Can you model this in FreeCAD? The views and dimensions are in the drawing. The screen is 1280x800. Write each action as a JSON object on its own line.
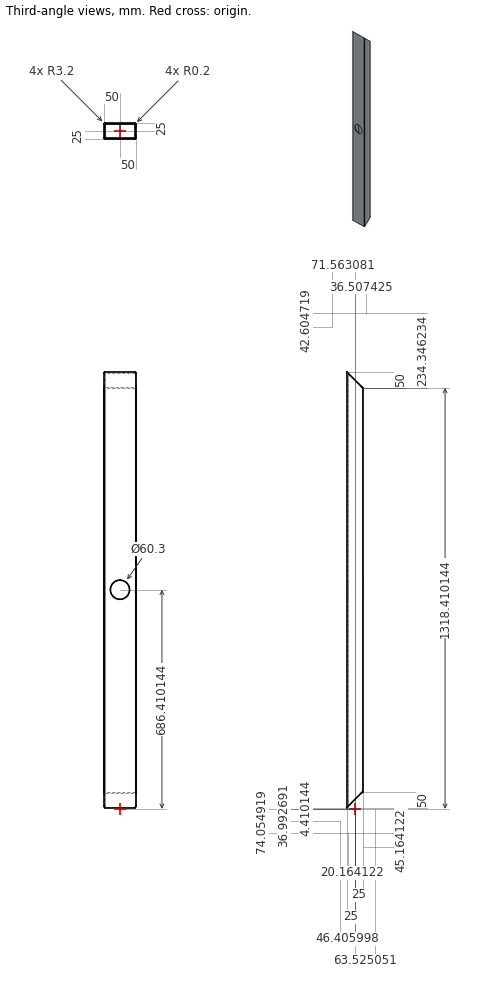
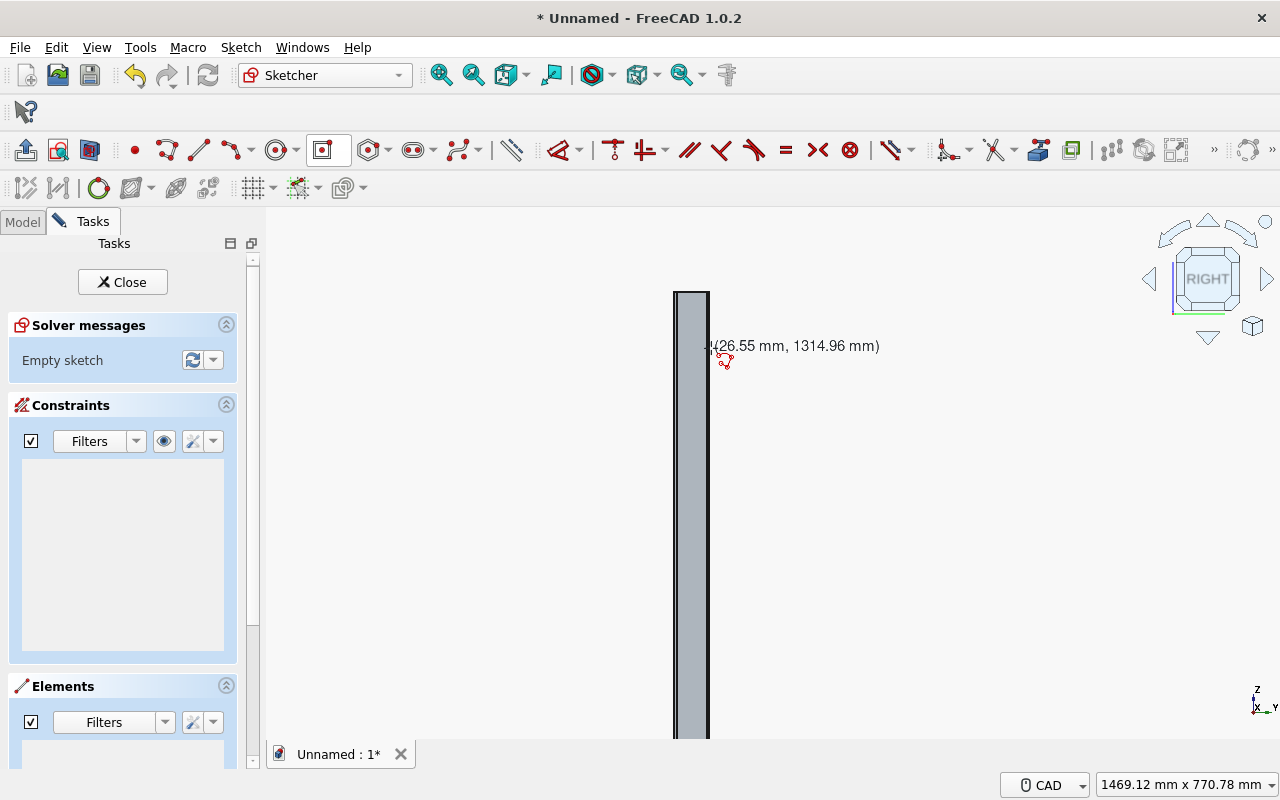
{"action": "left_click", "coordinate": [709, 348]}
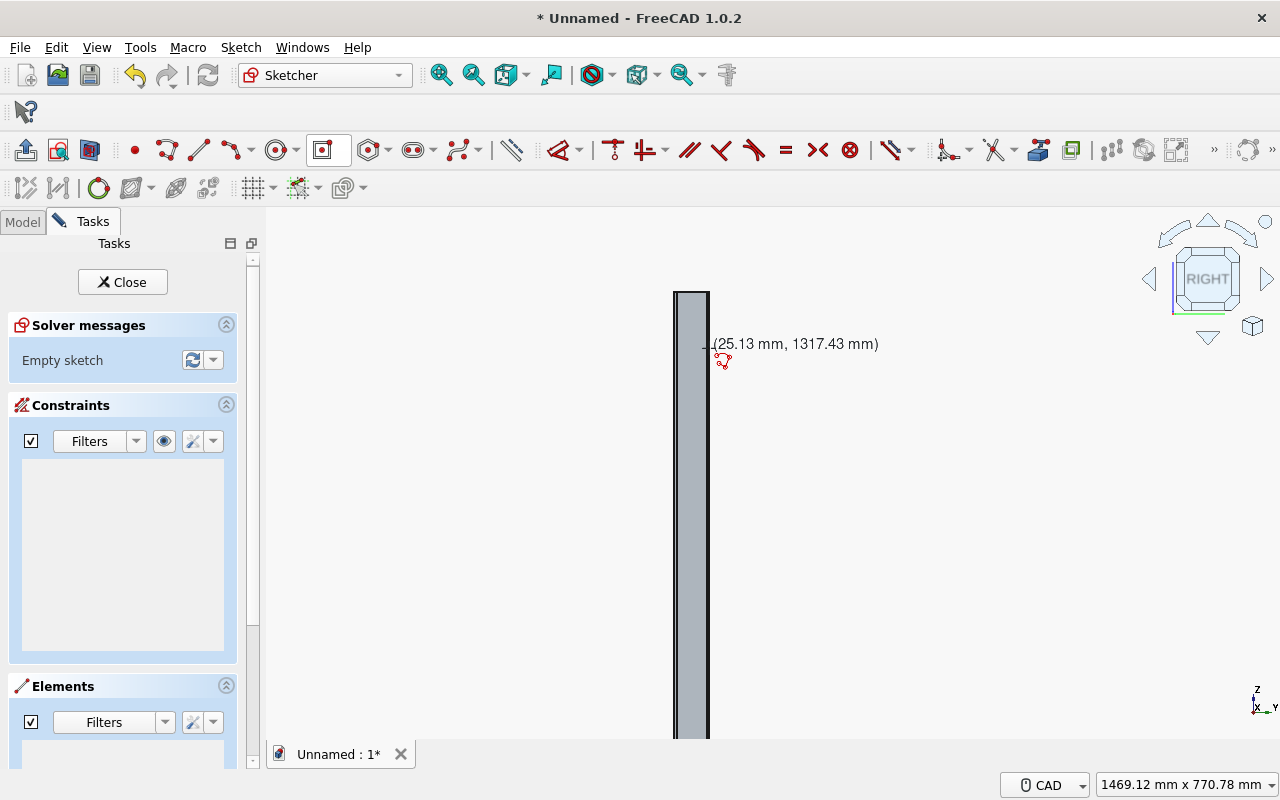
{"action": "scroll", "coordinate": [711, 348], "scroll_direction": "down", "scroll_amount": 6}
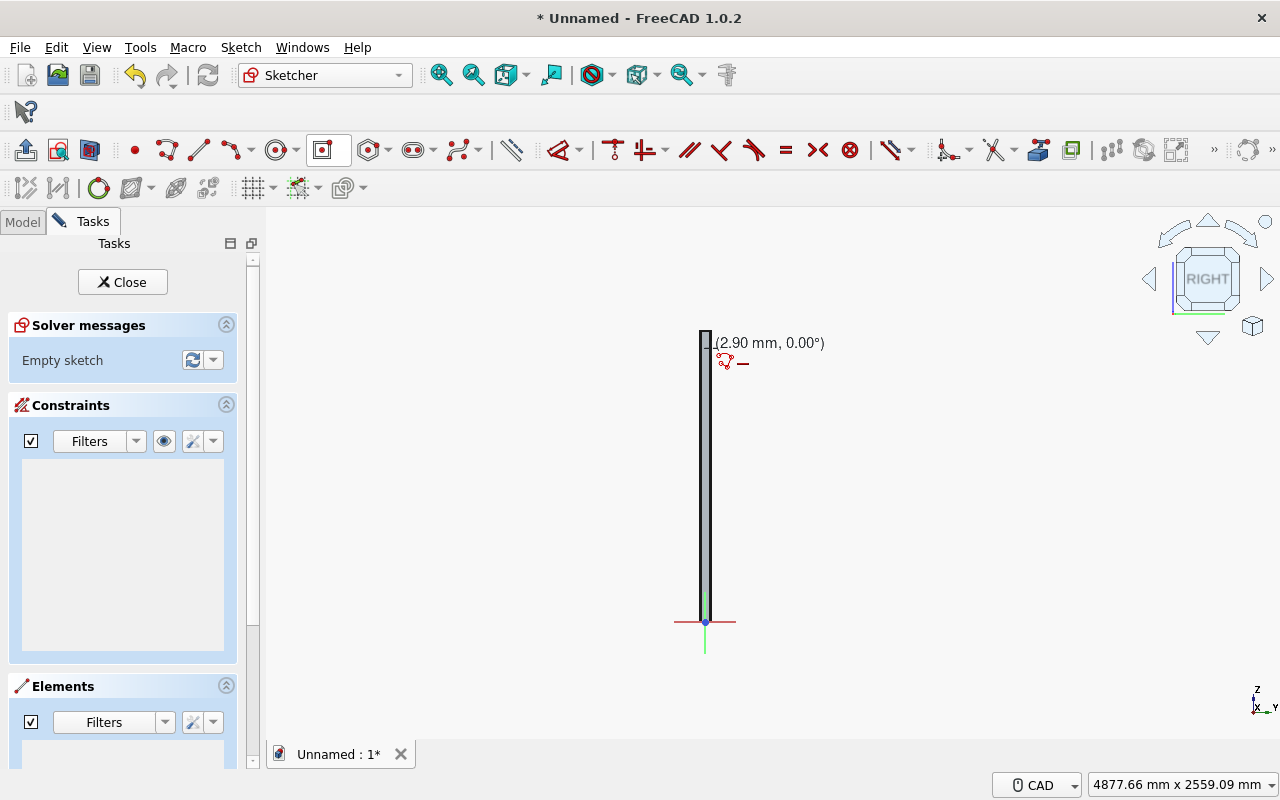
{"action": "scroll", "coordinate": [713, 300], "scroll_direction": "up", "scroll_amount": 4}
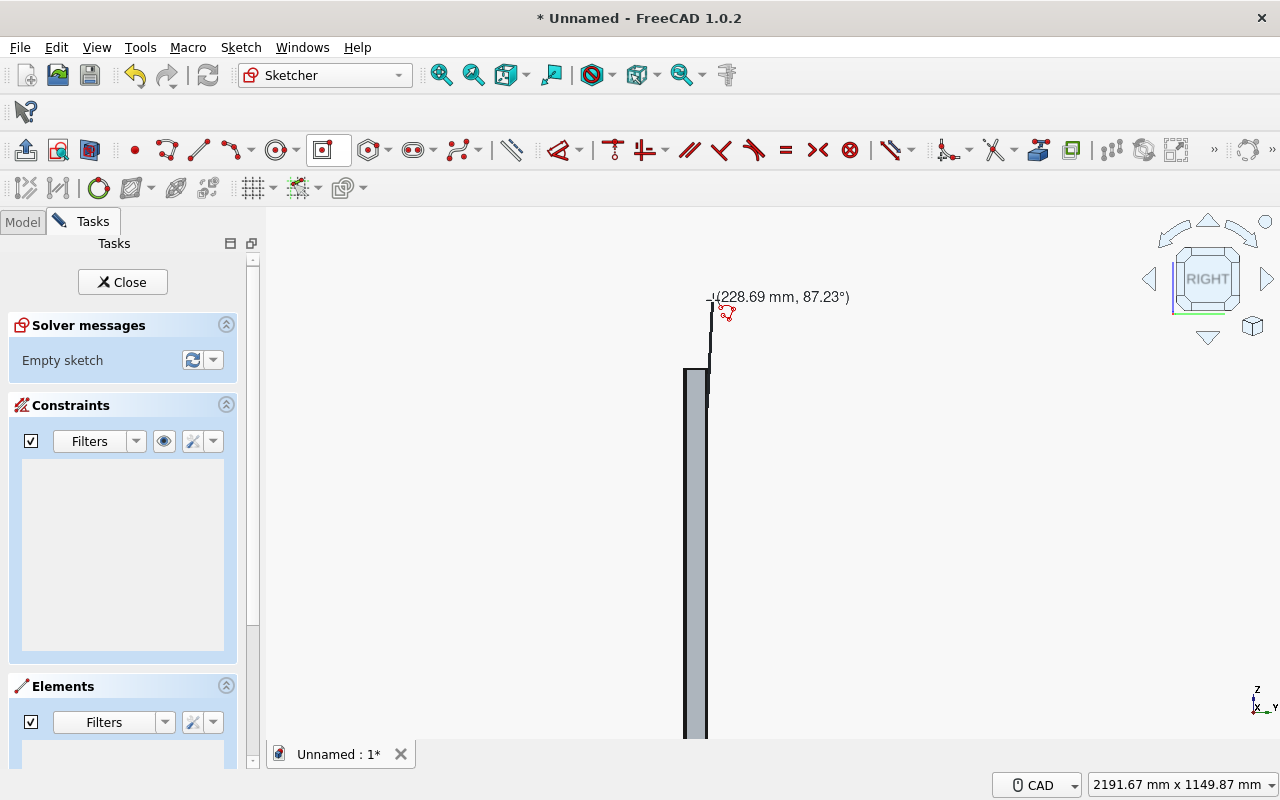
{"action": "left_click", "coordinate": [714, 299]}
{"action": "left_click", "coordinate": [663, 319]}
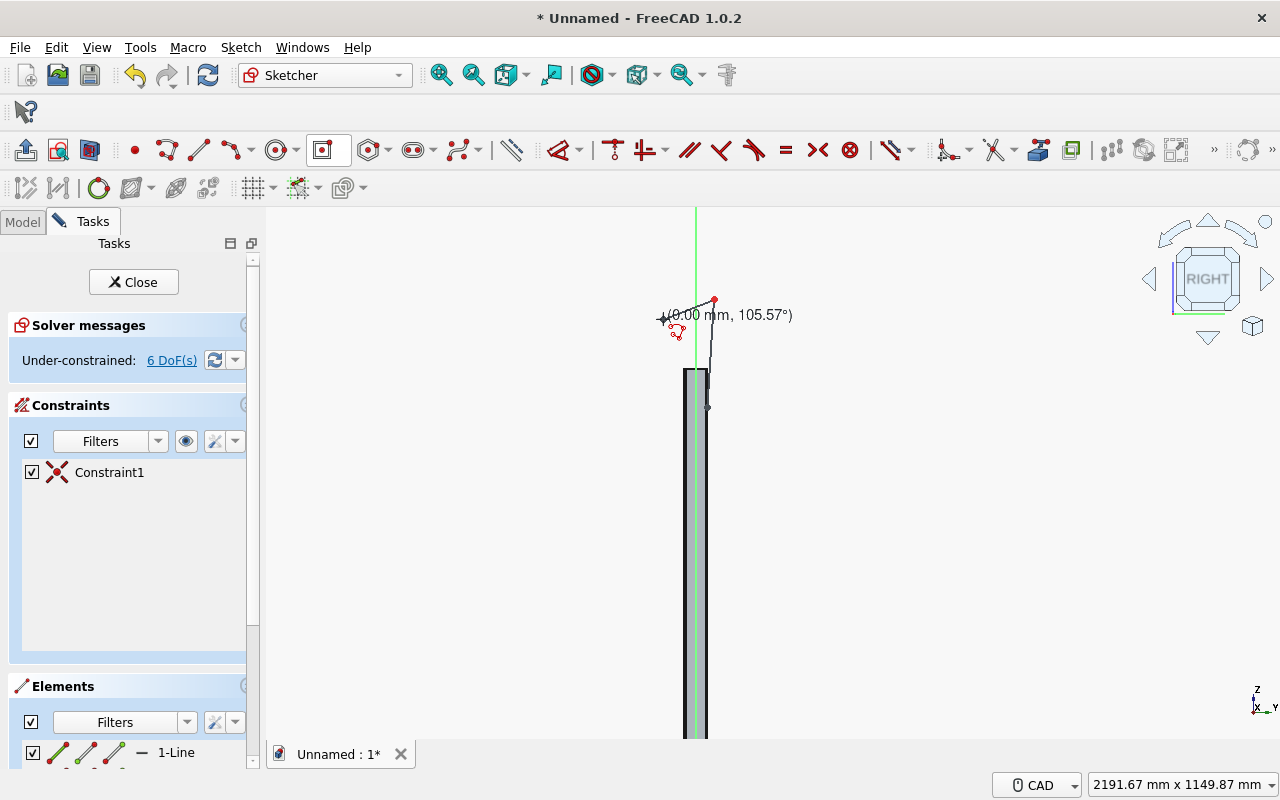
{"action": "scroll", "coordinate": [684, 384], "scroll_direction": "up", "scroll_amount": 2}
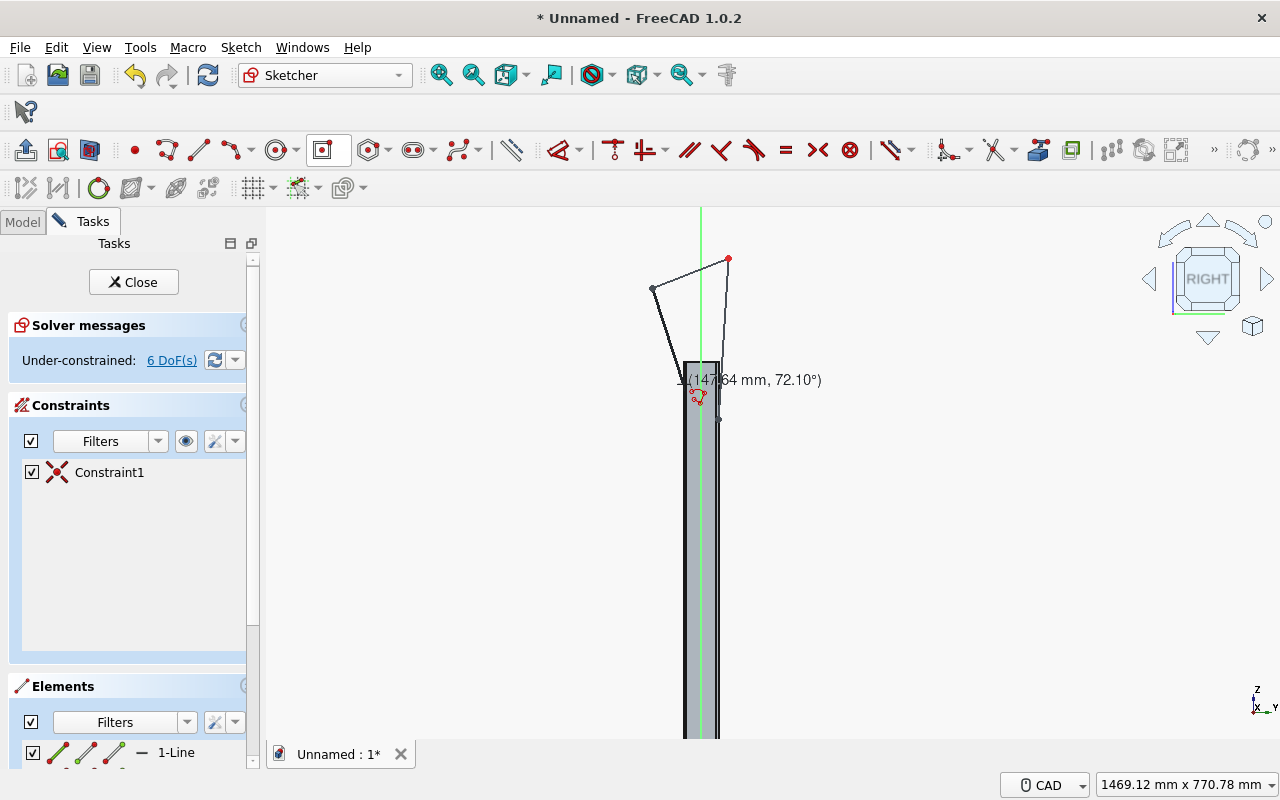
{"action": "left_click", "coordinate": [684, 384]}
{"action": "left_click", "coordinate": [719, 419]}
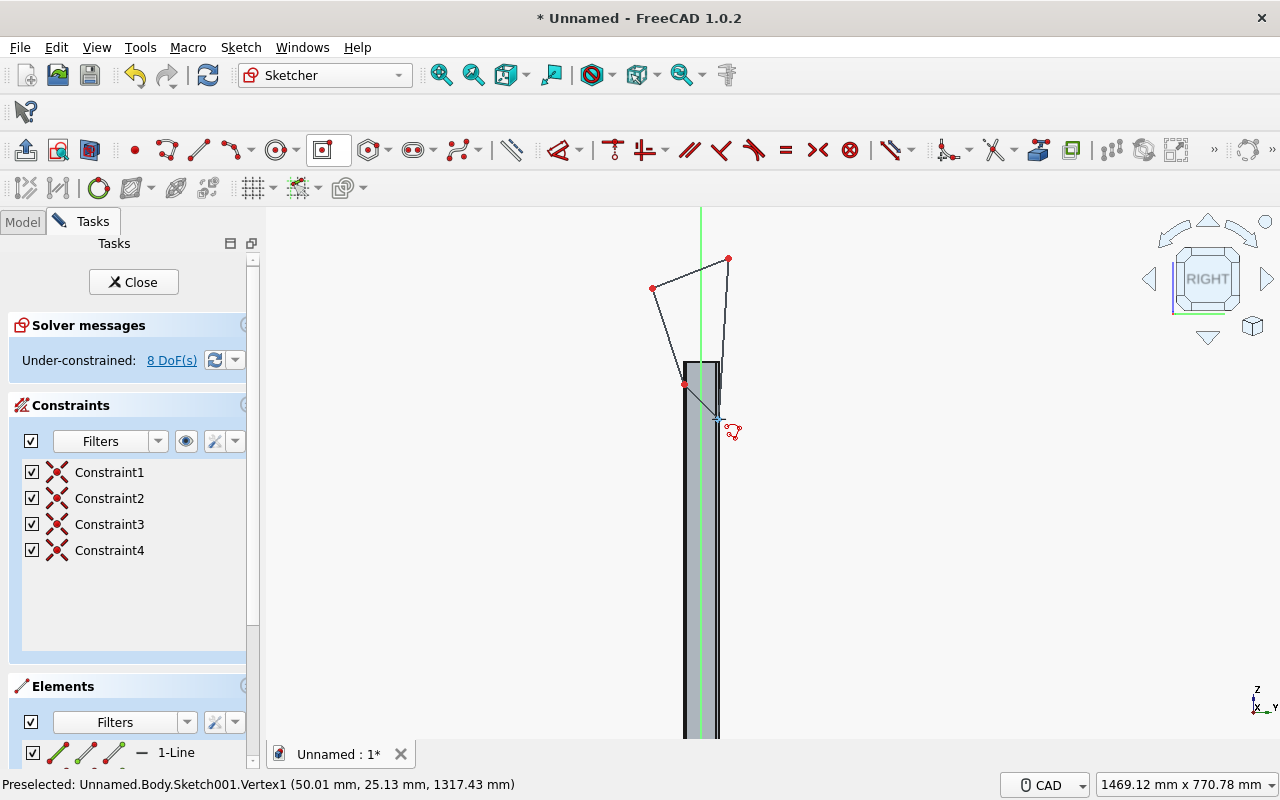
{"action": "scroll", "coordinate": [707, 318], "scroll_direction": "down", "scroll_amount": 6}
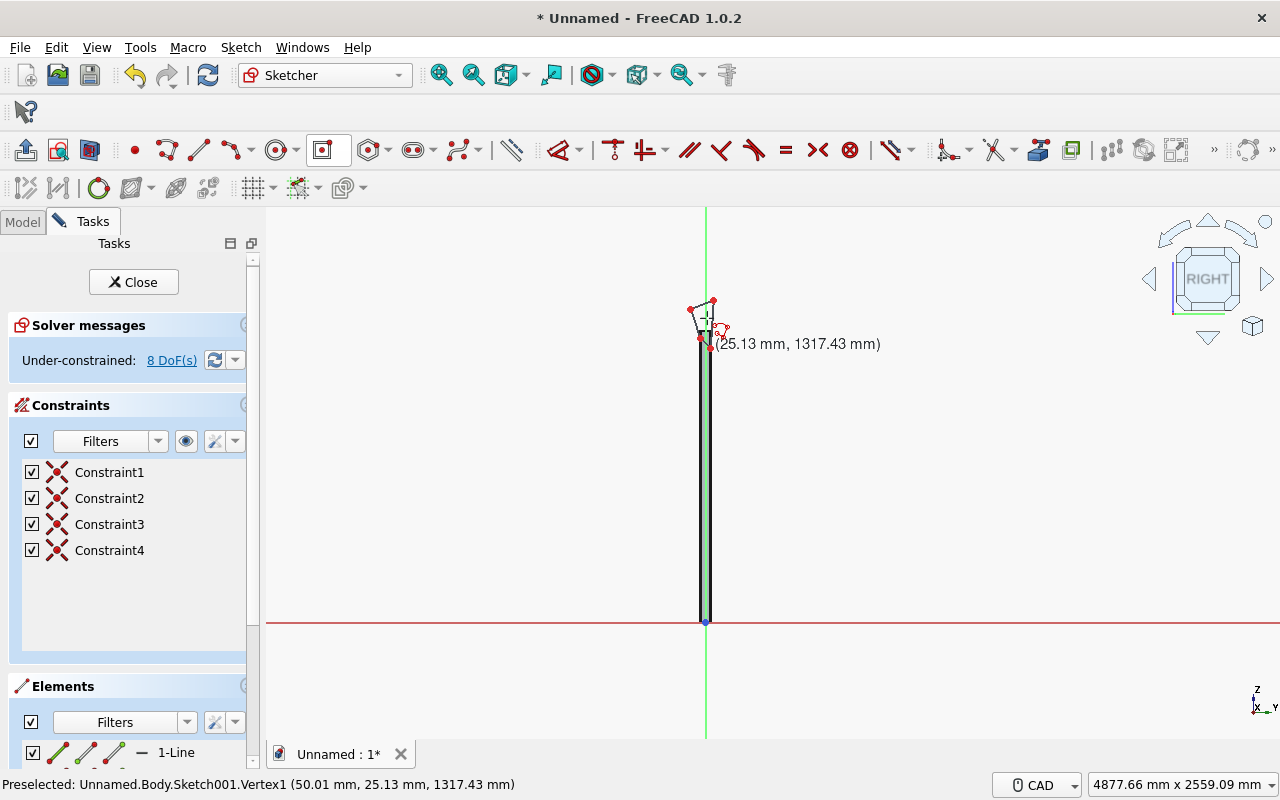
{"action": "scroll", "coordinate": [700, 622], "scroll_direction": "up", "scroll_amount": 15}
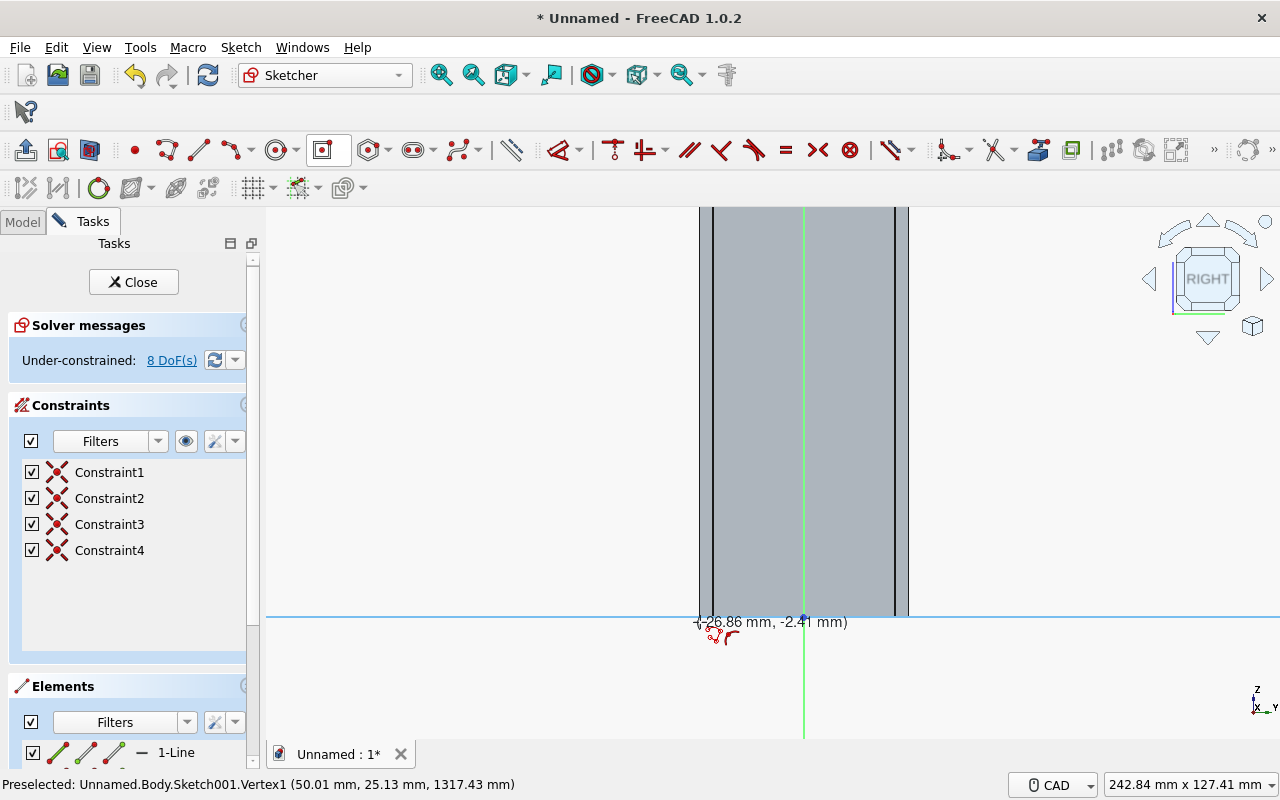
{"action": "left_click", "coordinate": [700, 599]}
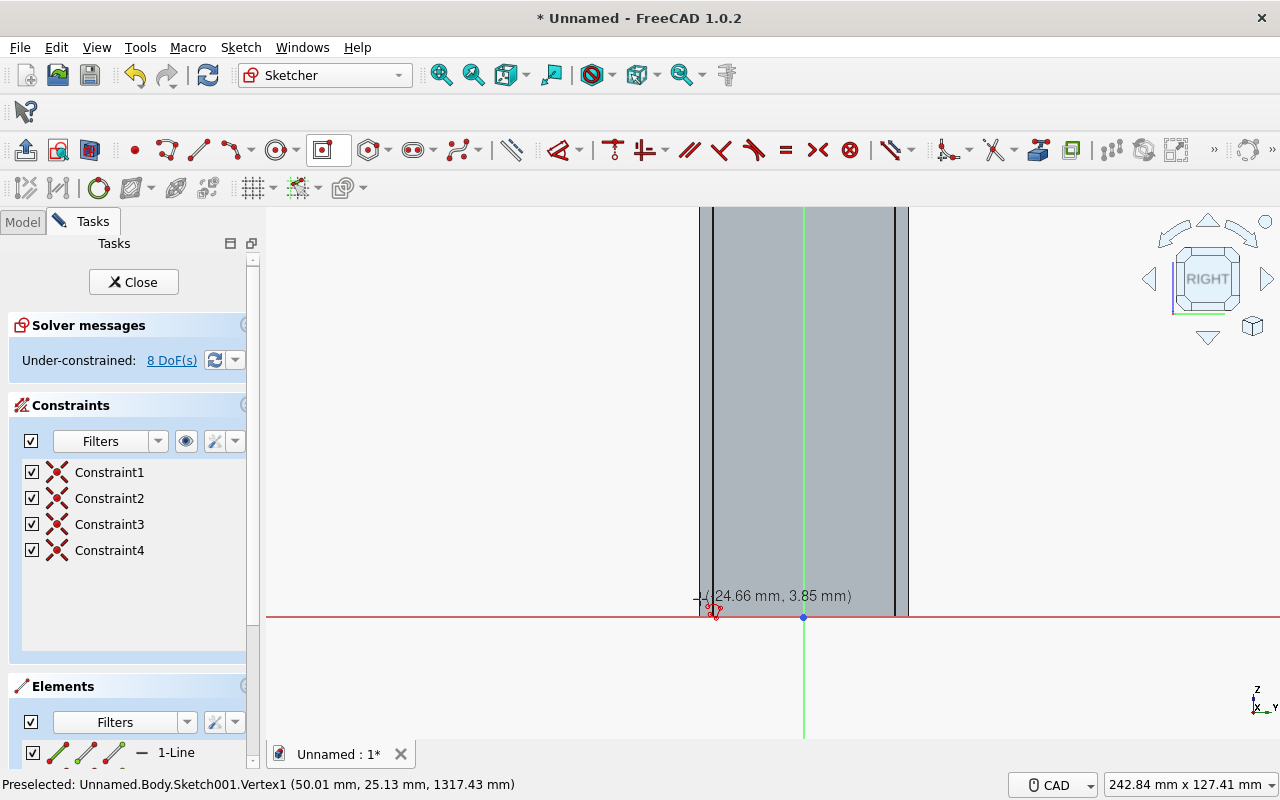
{"action": "scroll", "coordinate": [700, 622], "scroll_direction": "down", "scroll_amount": 15}